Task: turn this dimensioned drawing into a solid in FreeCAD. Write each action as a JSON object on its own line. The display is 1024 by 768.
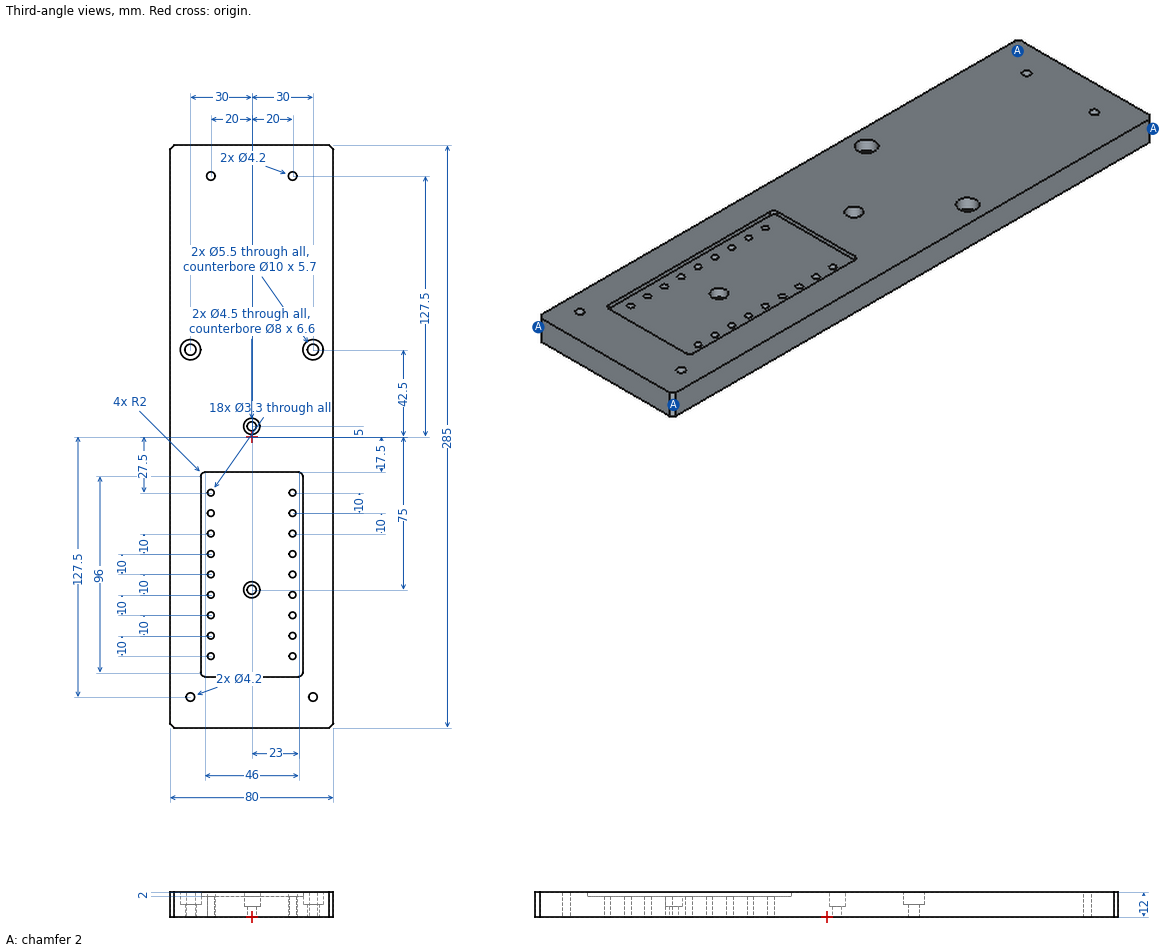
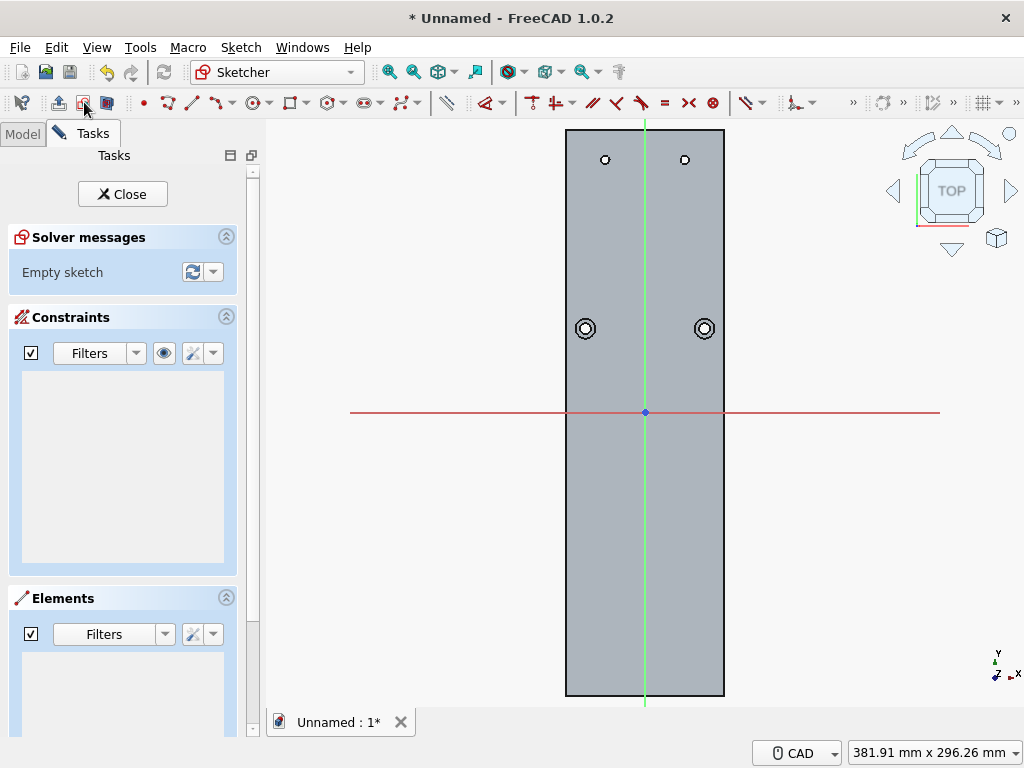
{"action": "scroll", "coordinate": [784, 679], "scroll_direction": "up", "scroll_amount": 2}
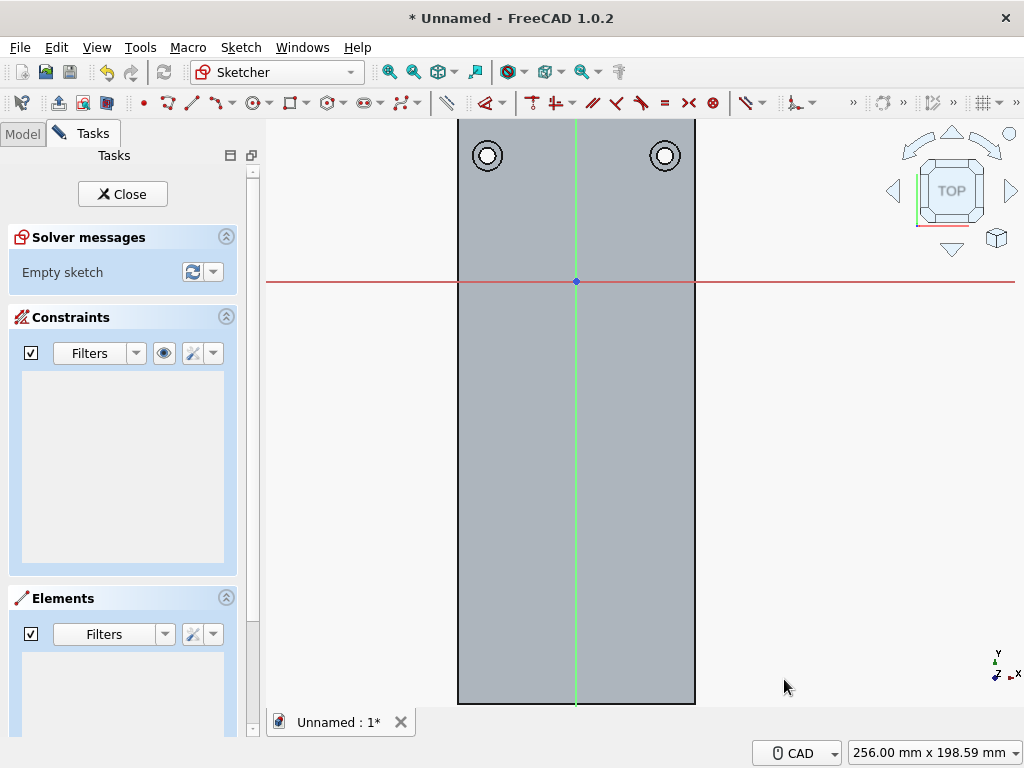
{"action": "key", "text": "g l"}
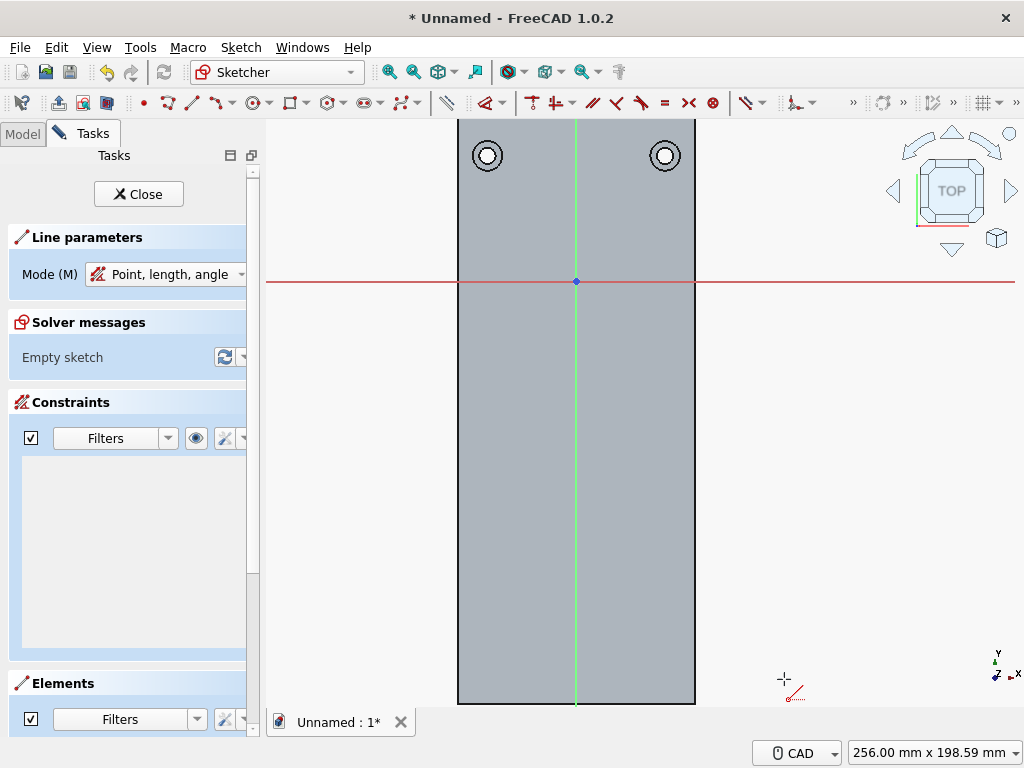
{"action": "left_click", "coordinate": [644, 334]}
{"action": "left_click", "coordinate": [508, 334]}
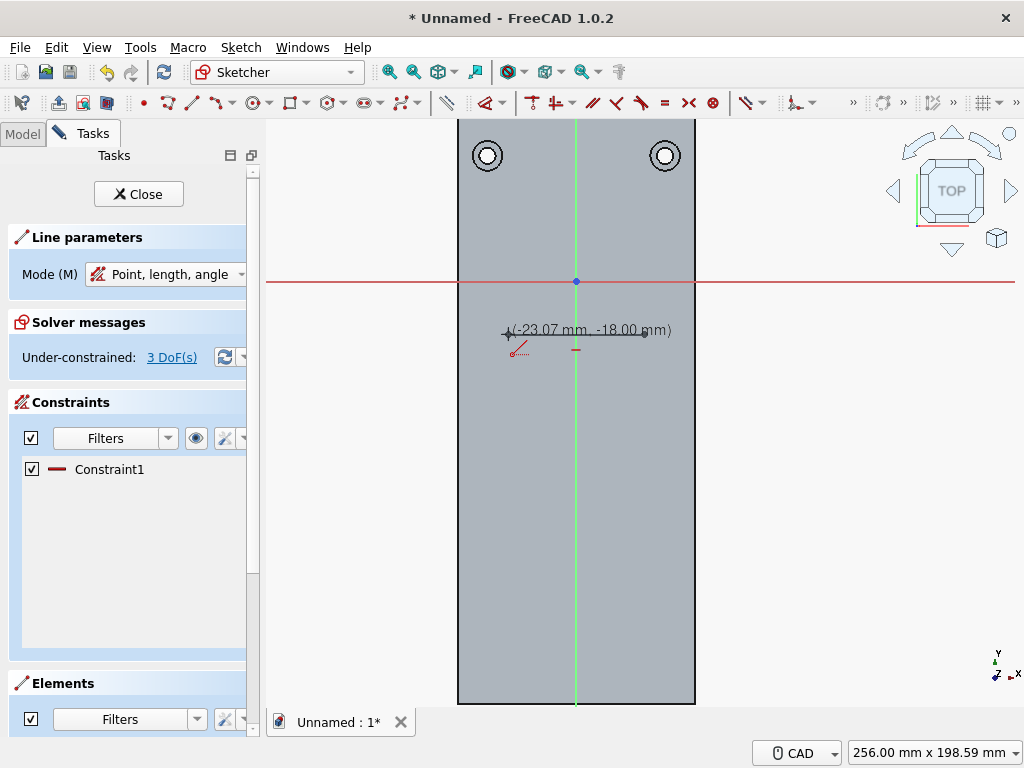
{"action": "scroll", "coordinate": [502, 339], "scroll_direction": "up", "scroll_amount": 4}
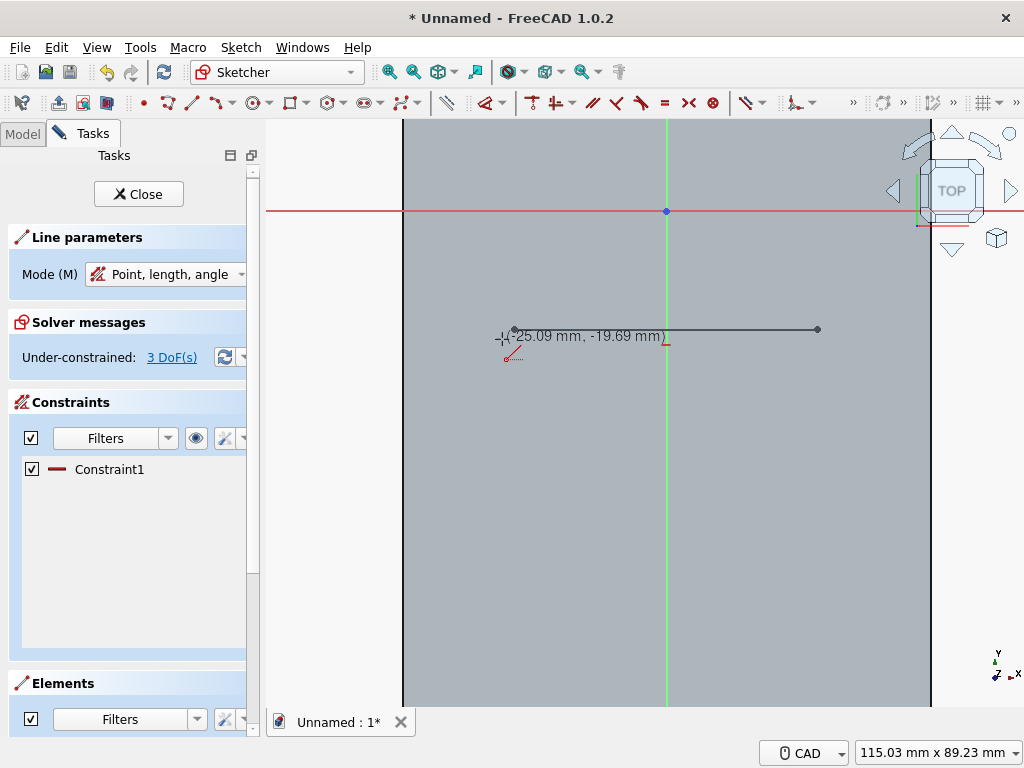
{"action": "left_click", "coordinate": [502, 340]}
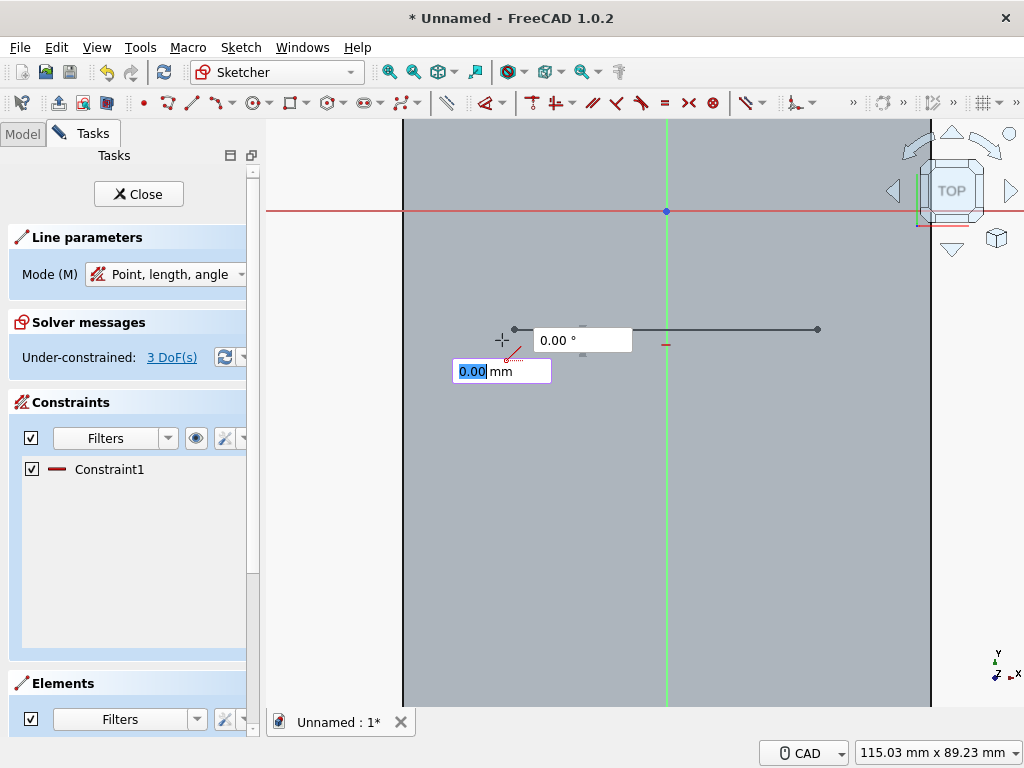
{"action": "scroll", "coordinate": [503, 262], "scroll_direction": "down", "scroll_amount": 4}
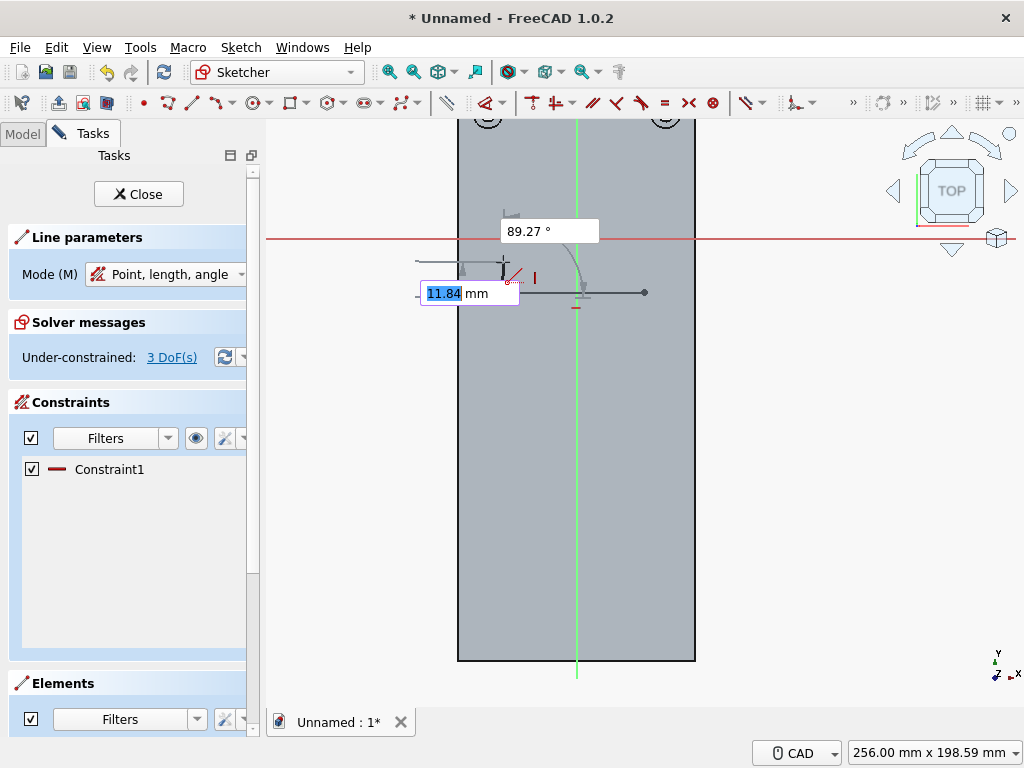
{"action": "left_click", "coordinate": [503, 581]}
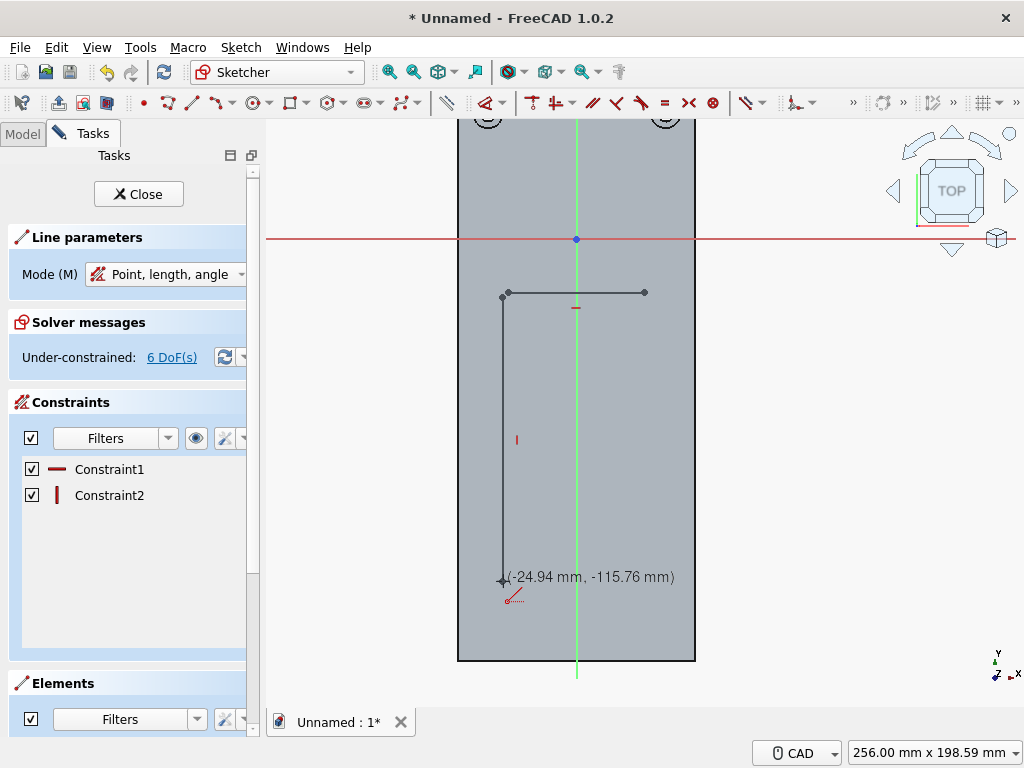
{"action": "scroll", "coordinate": [509, 587], "scroll_direction": "up", "scroll_amount": 4}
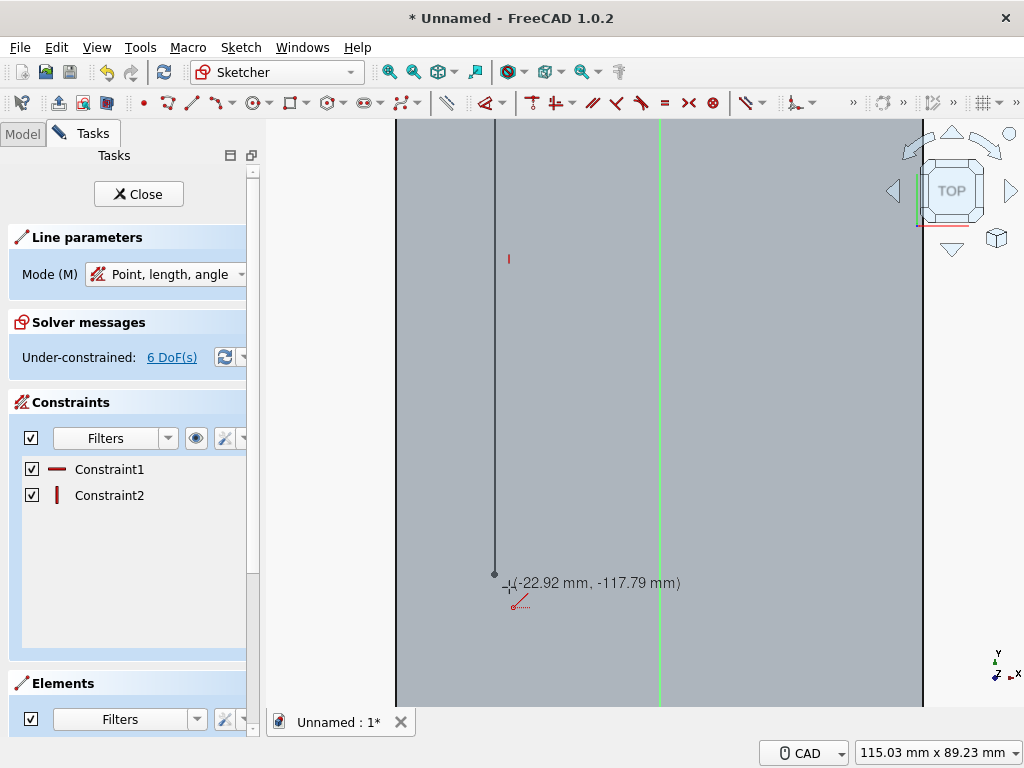
{"action": "left_click", "coordinate": [508, 586]}
{"action": "left_click", "coordinate": [811, 586]}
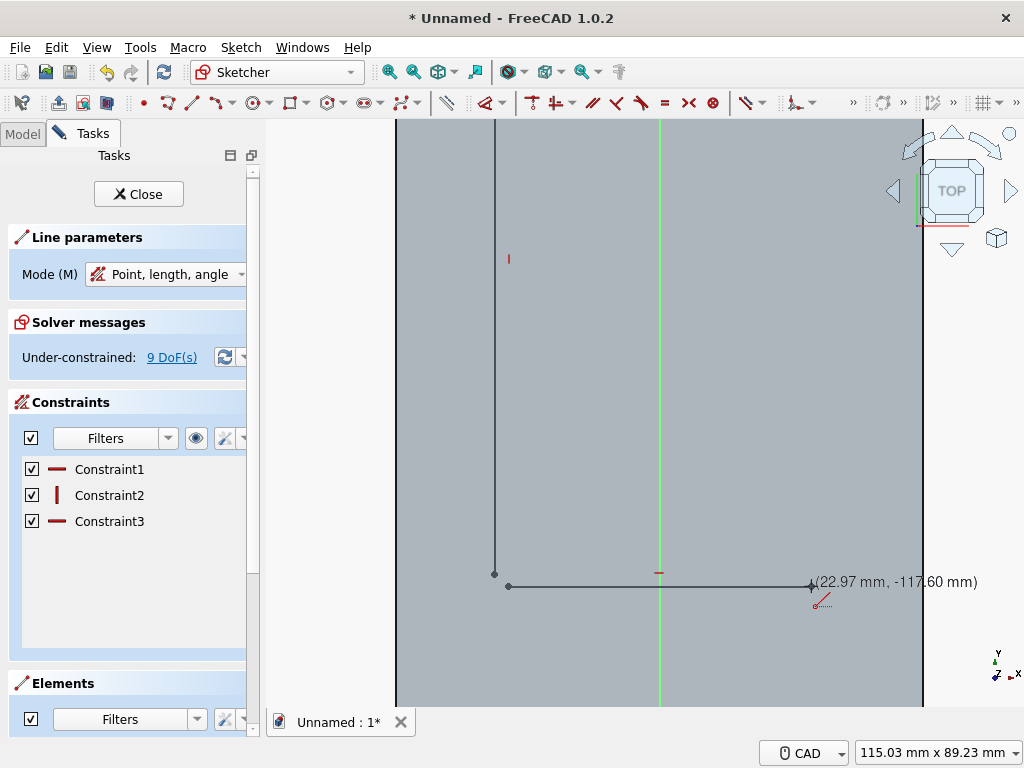
{"action": "left_click", "coordinate": [824, 573]}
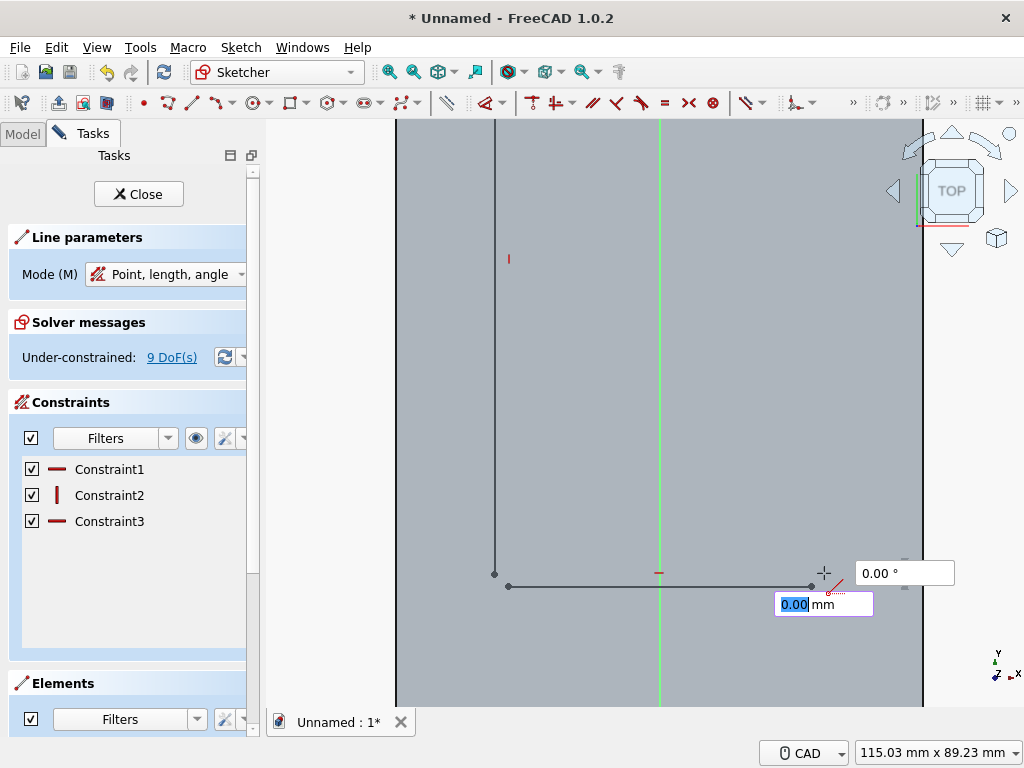
{"action": "scroll", "coordinate": [509, 587], "scroll_direction": "down", "scroll_amount": 4}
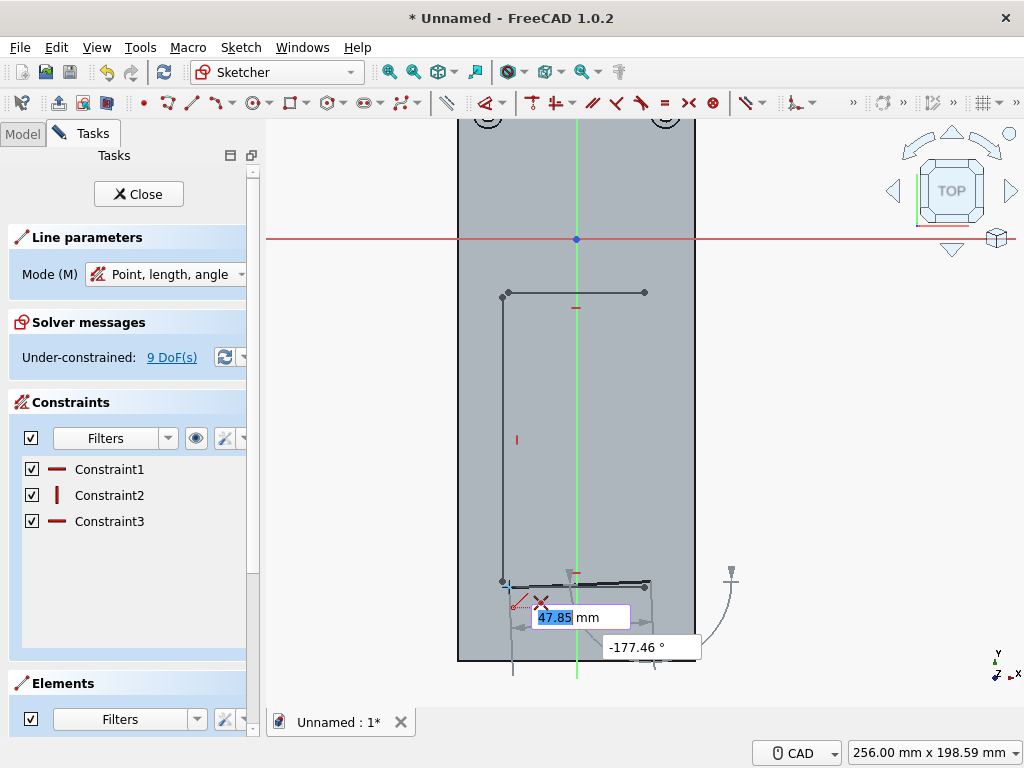
{"action": "scroll", "coordinate": [651, 297], "scroll_direction": "up", "scroll_amount": 4}